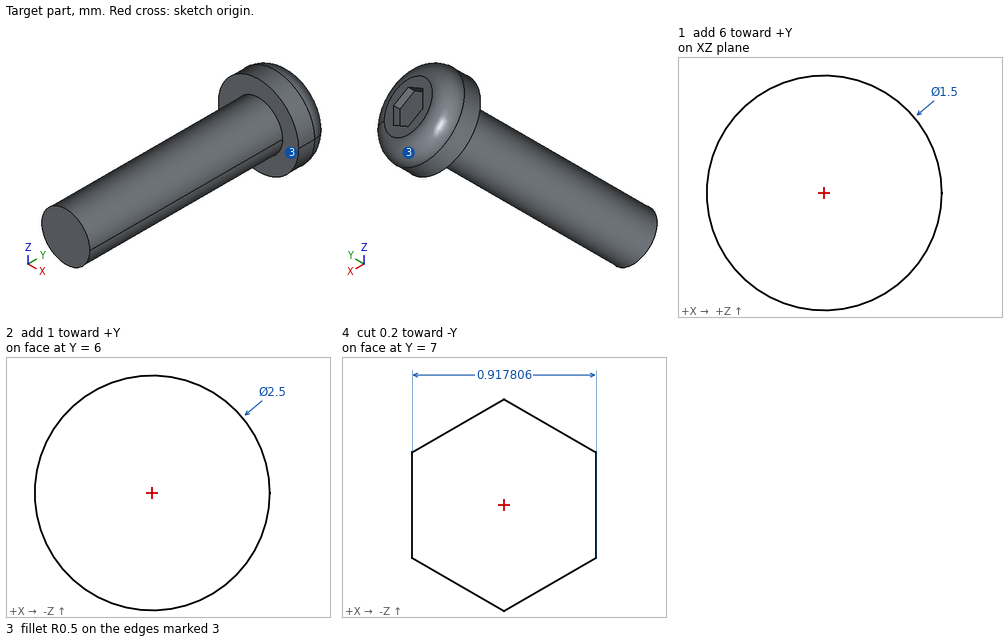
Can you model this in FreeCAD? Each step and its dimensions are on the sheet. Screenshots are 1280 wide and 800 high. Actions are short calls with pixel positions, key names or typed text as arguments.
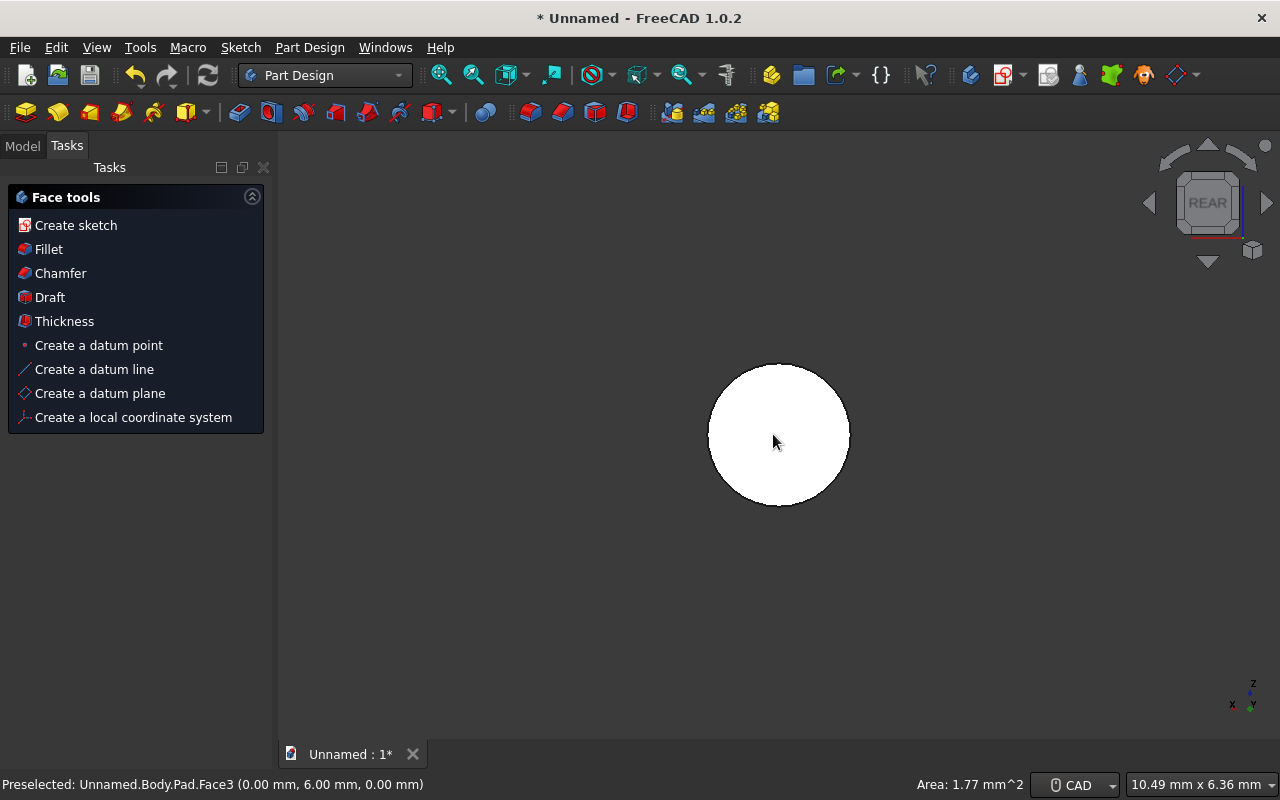
click(1004, 76)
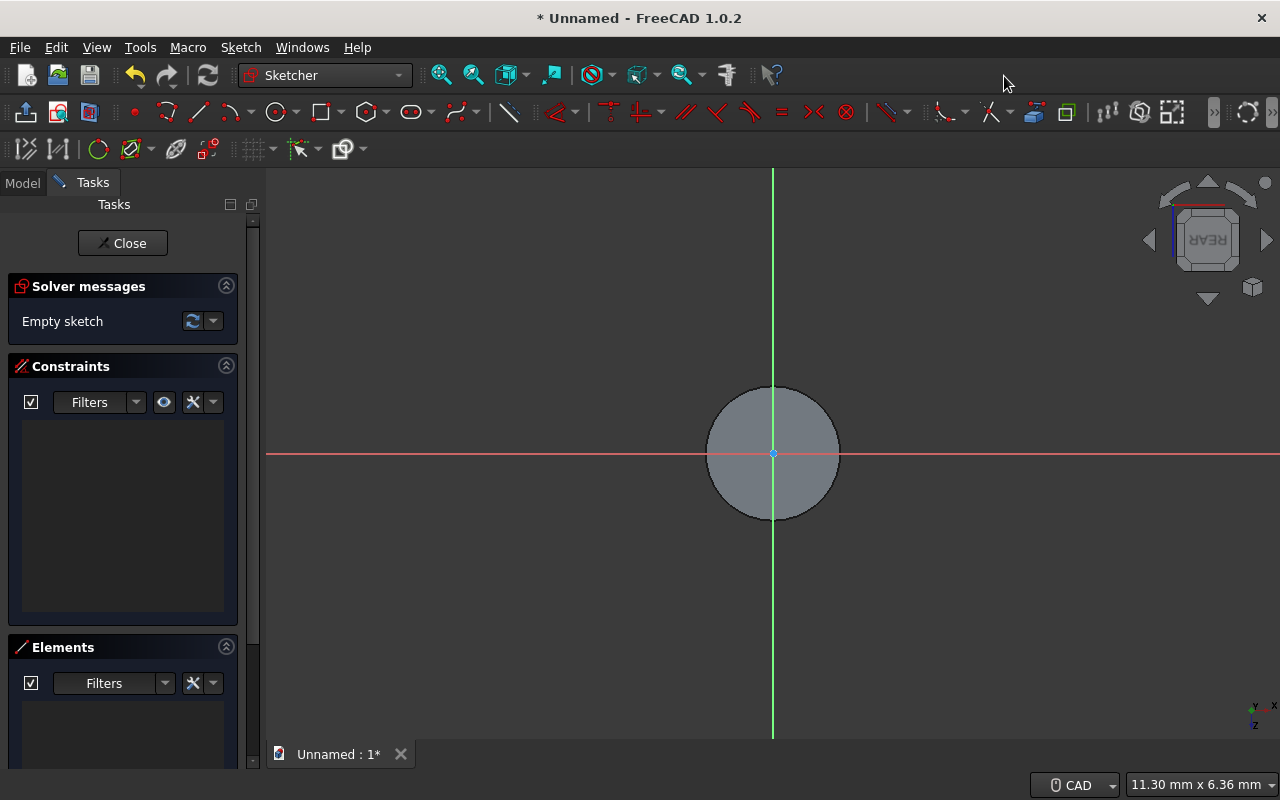
scroll(912, 453, up, 2)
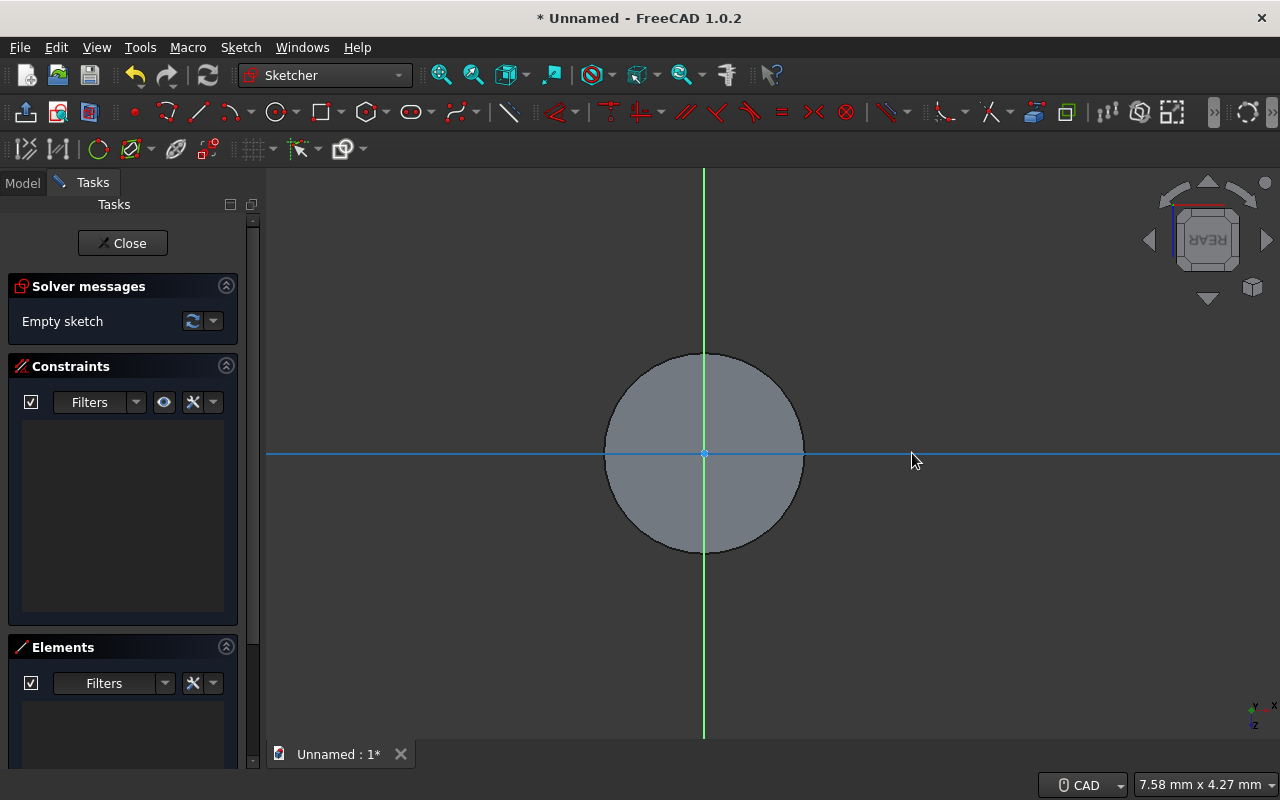
key(g)
key(c)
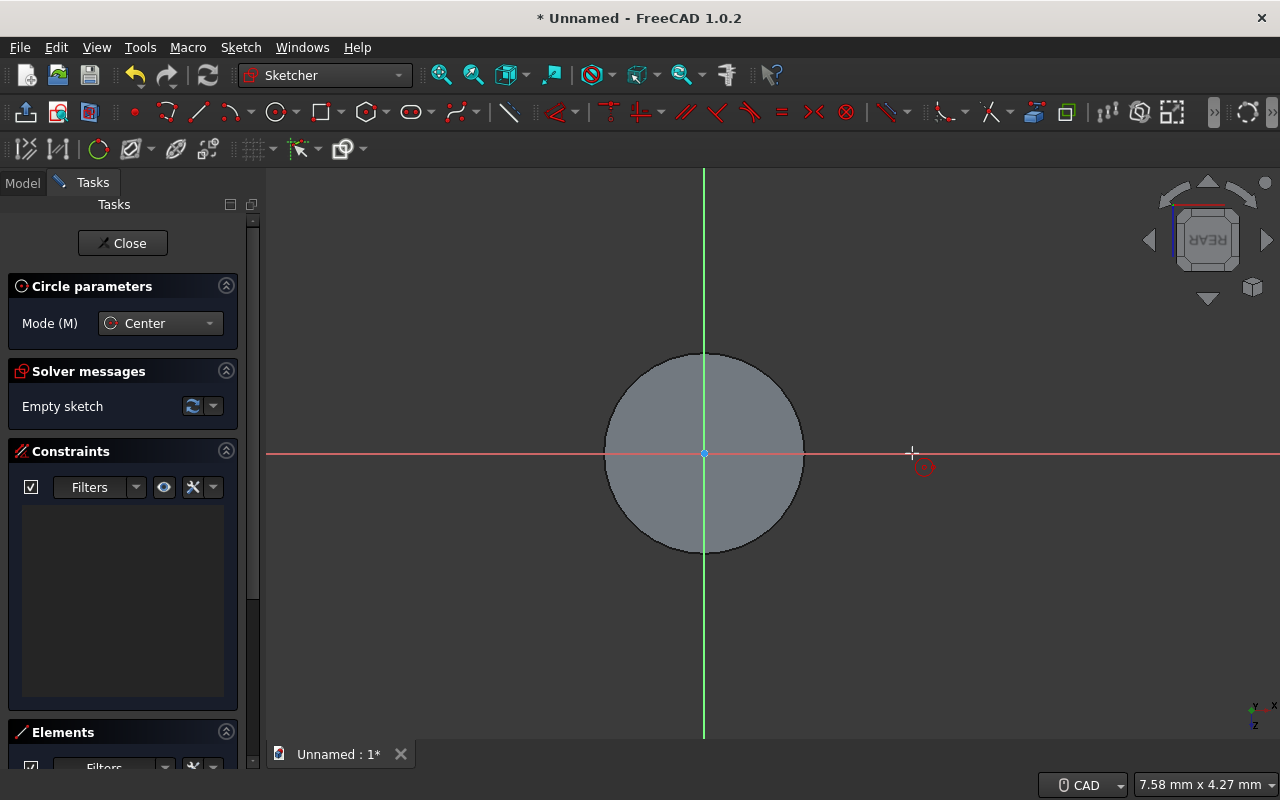
click(704, 453)
click(823, 335)
key(Escape)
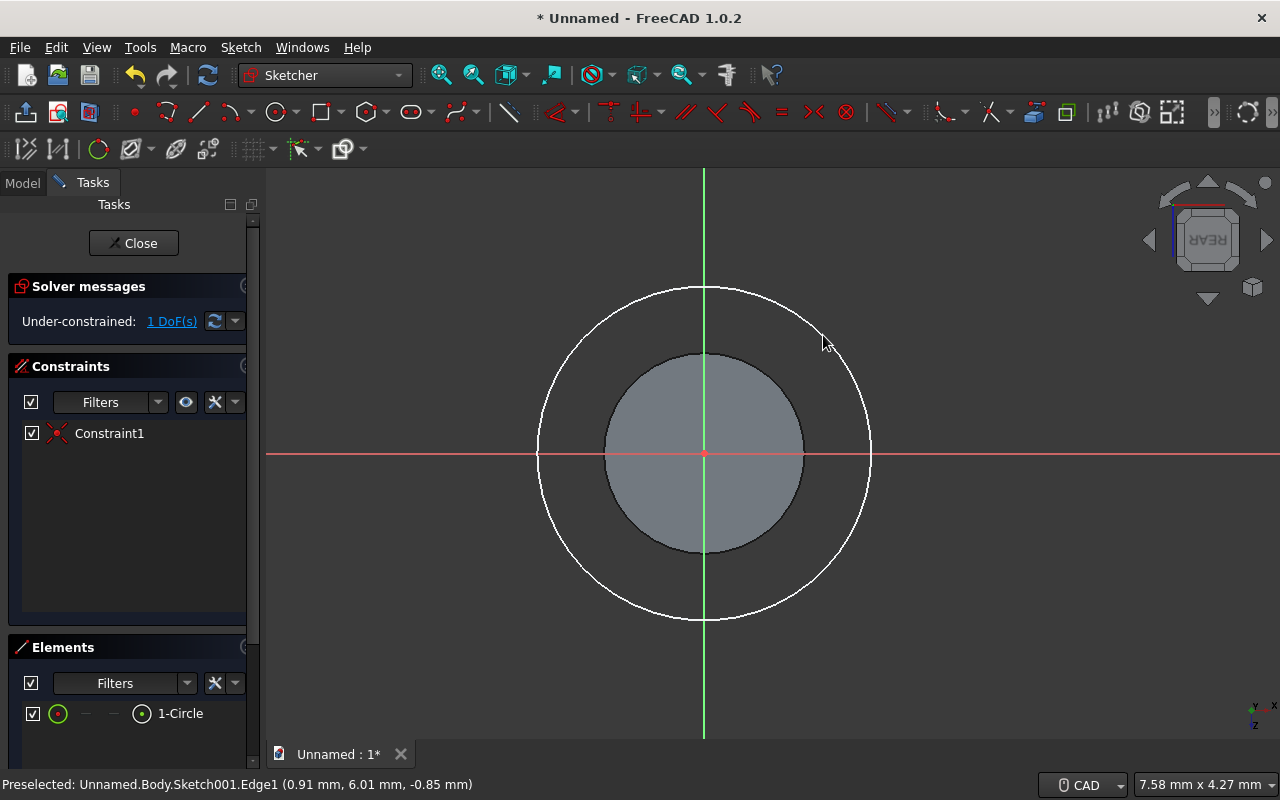
click(822, 335)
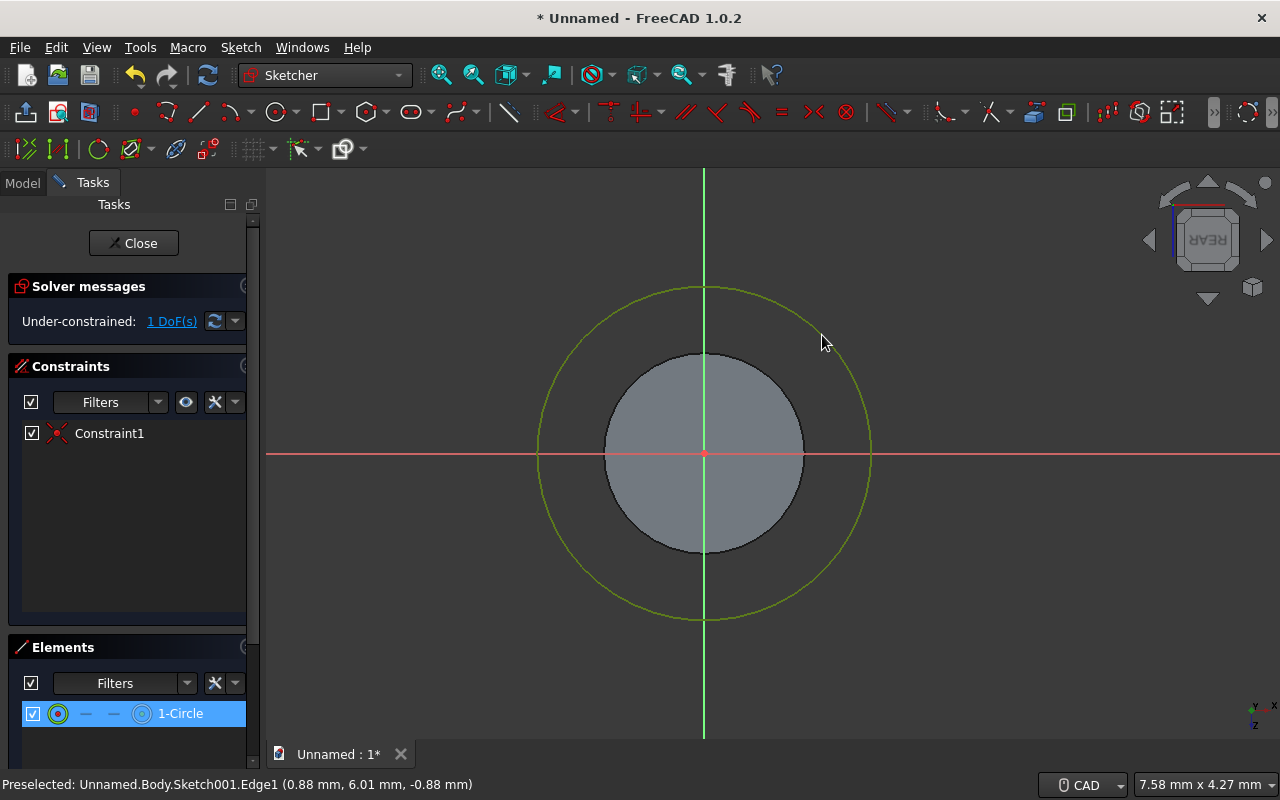
key(k)
key(o)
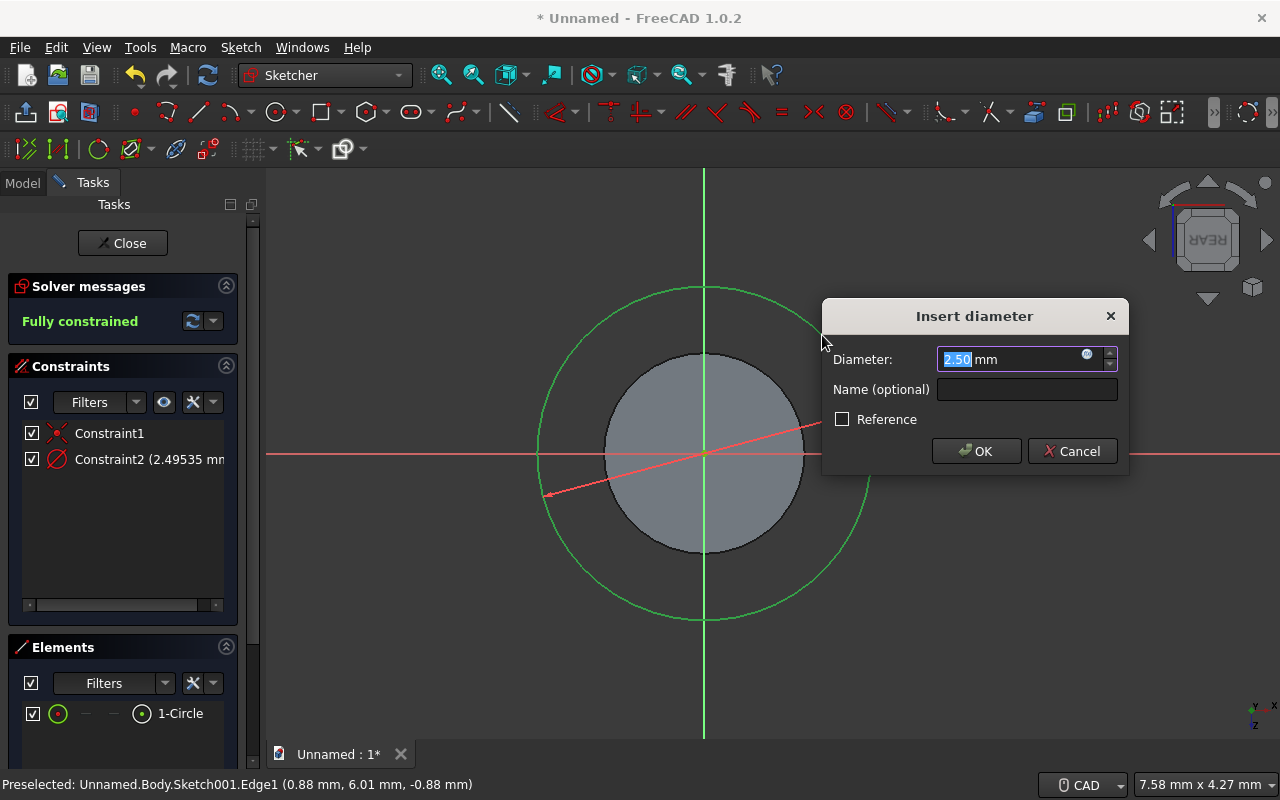
text(2.5)
key(Return)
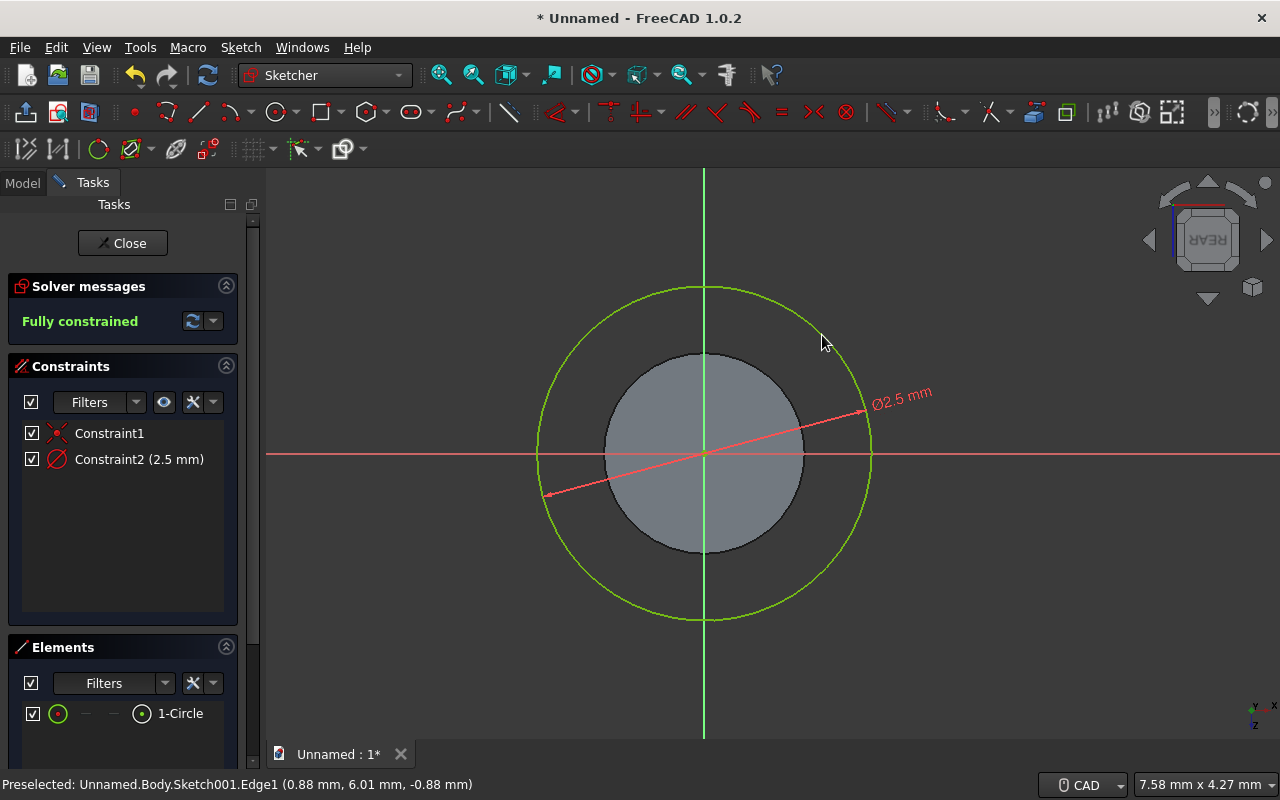
click(123, 243)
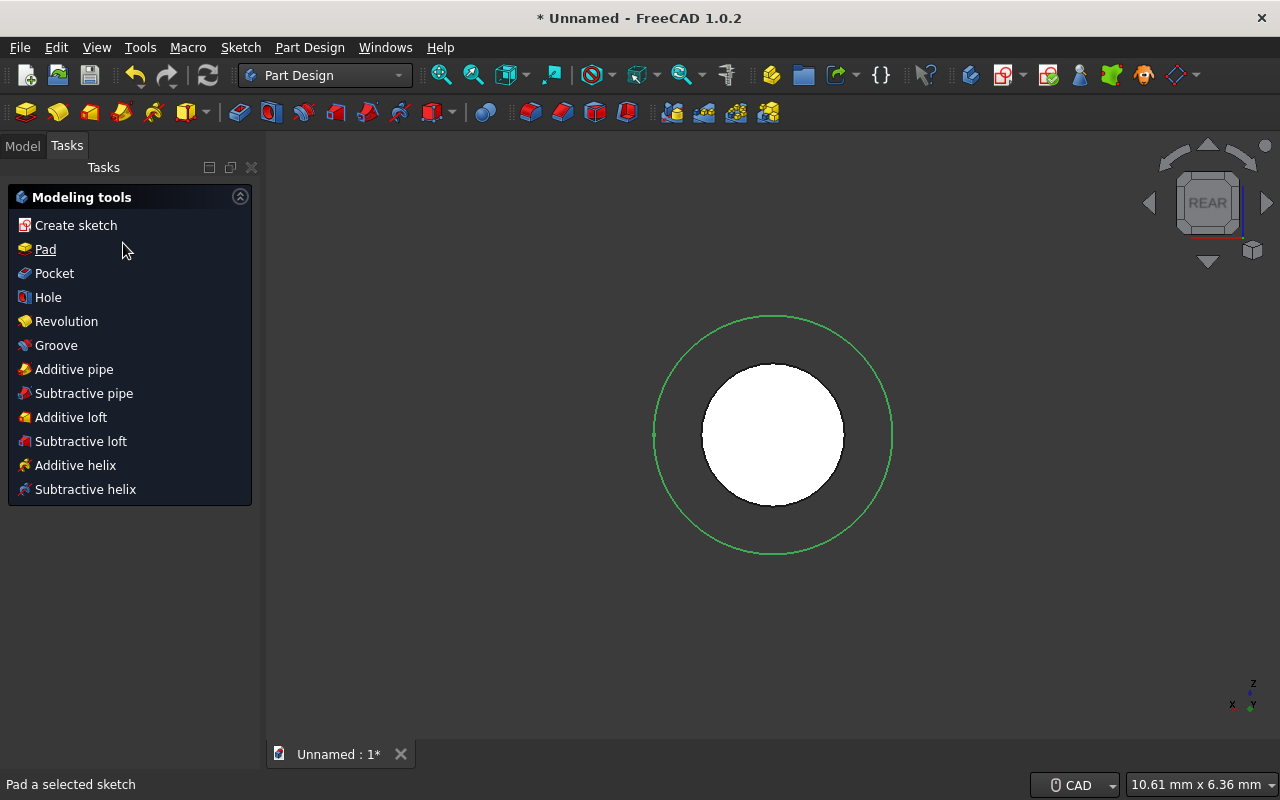
click(26, 112)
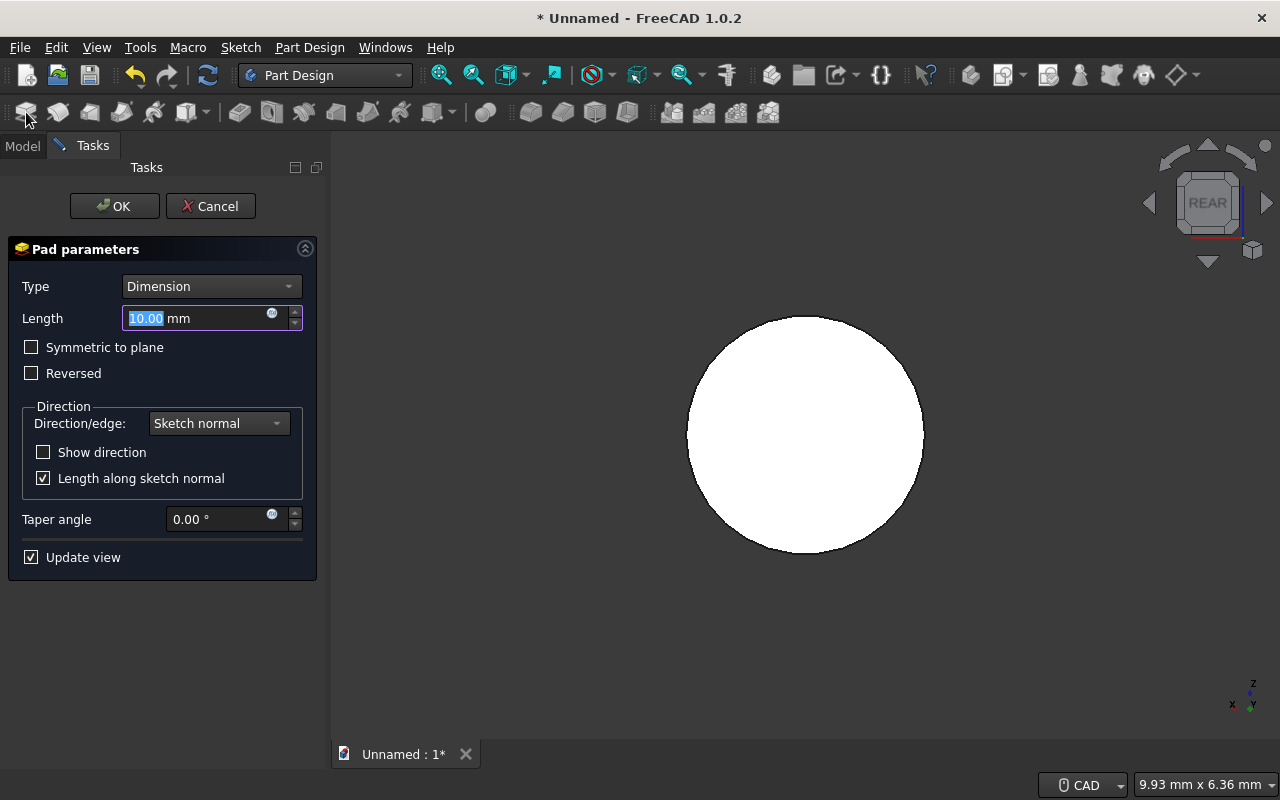
text(1)
key(Tab)